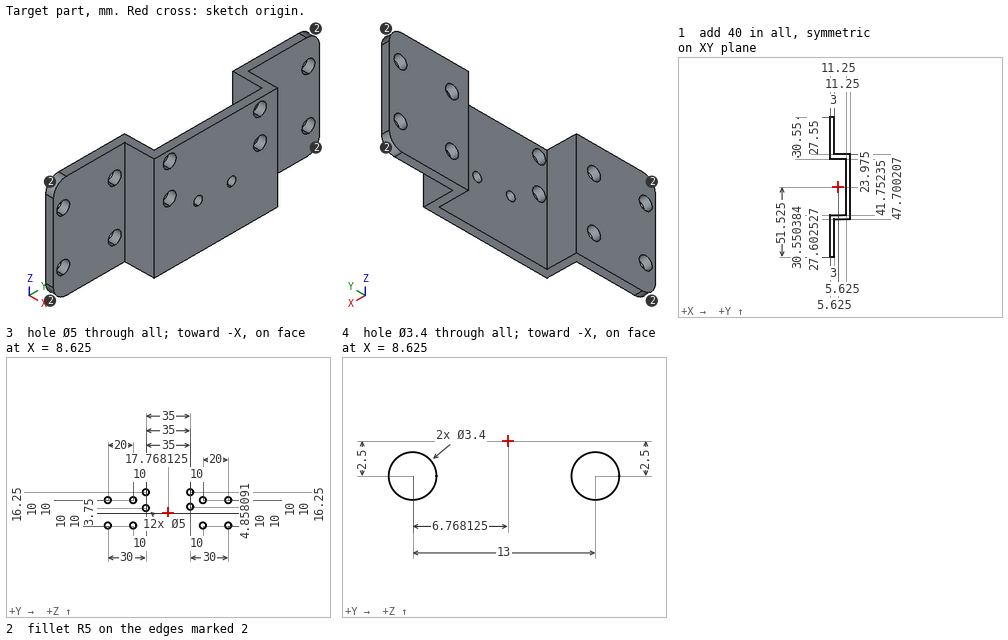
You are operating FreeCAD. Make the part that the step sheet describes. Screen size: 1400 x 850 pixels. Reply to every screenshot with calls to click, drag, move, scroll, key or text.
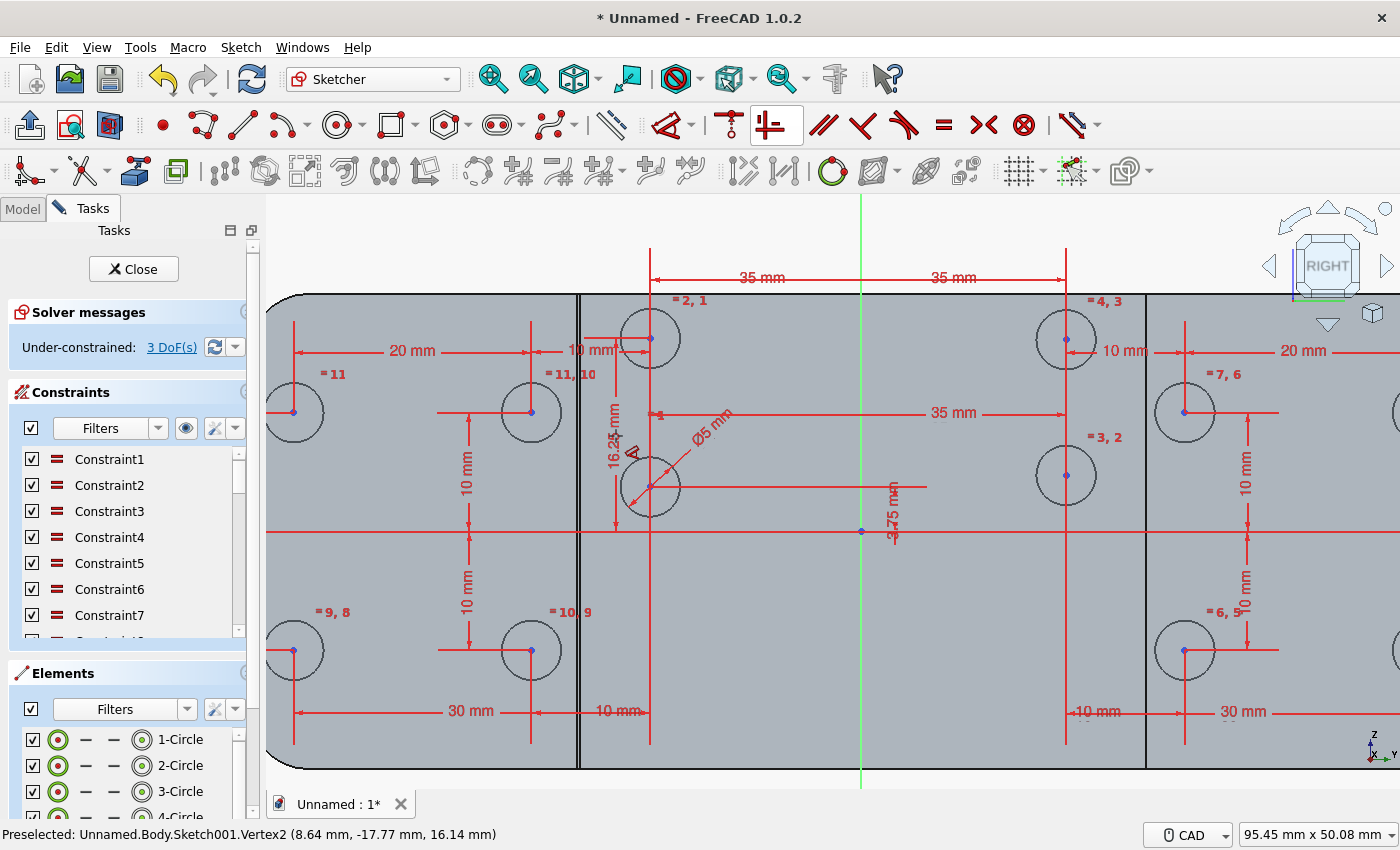
click(1066, 340)
click(1100, 436)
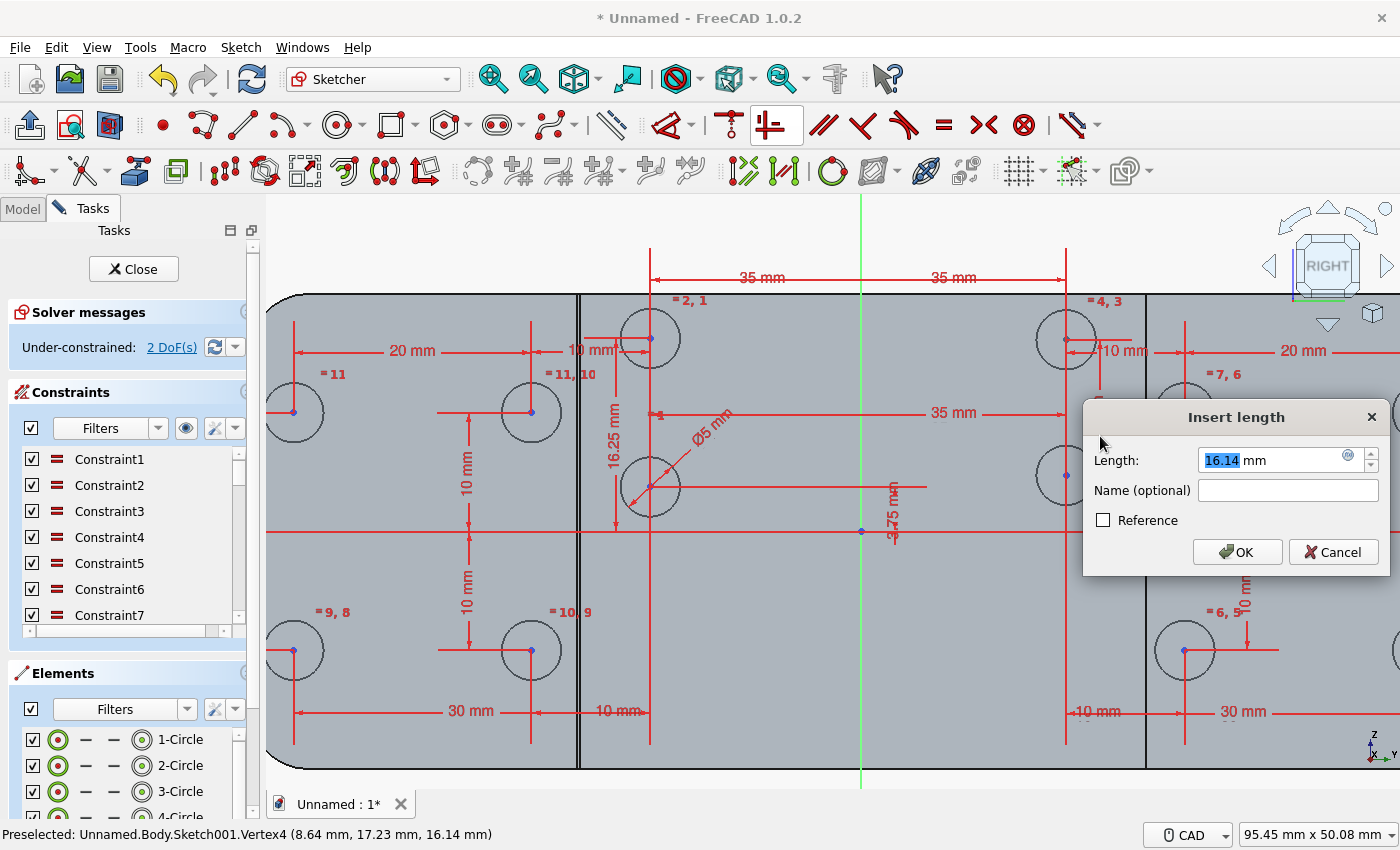
text(16.25)
key(Return)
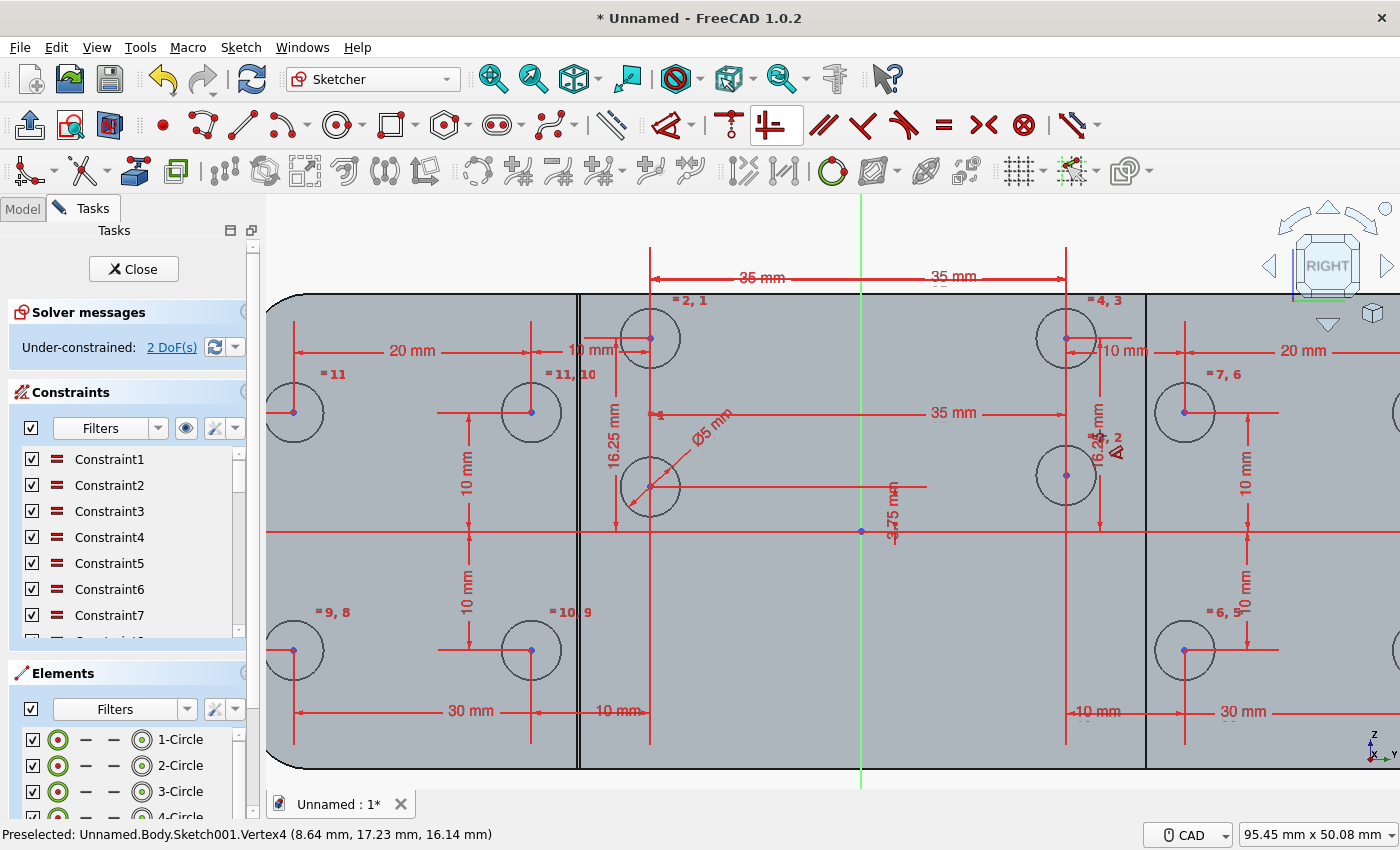
click(1066, 475)
click(1100, 503)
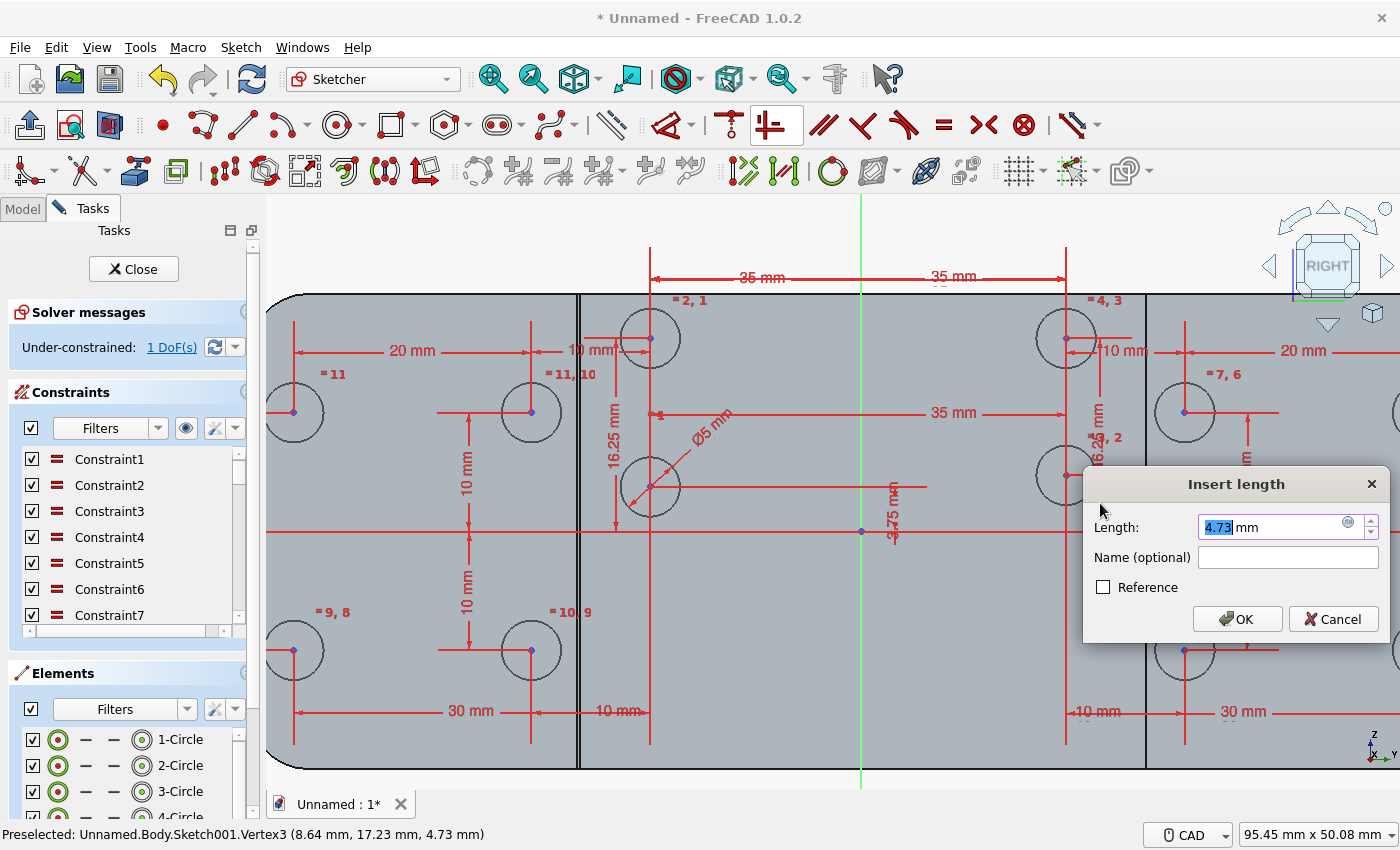
text(4.858091)
key(Return)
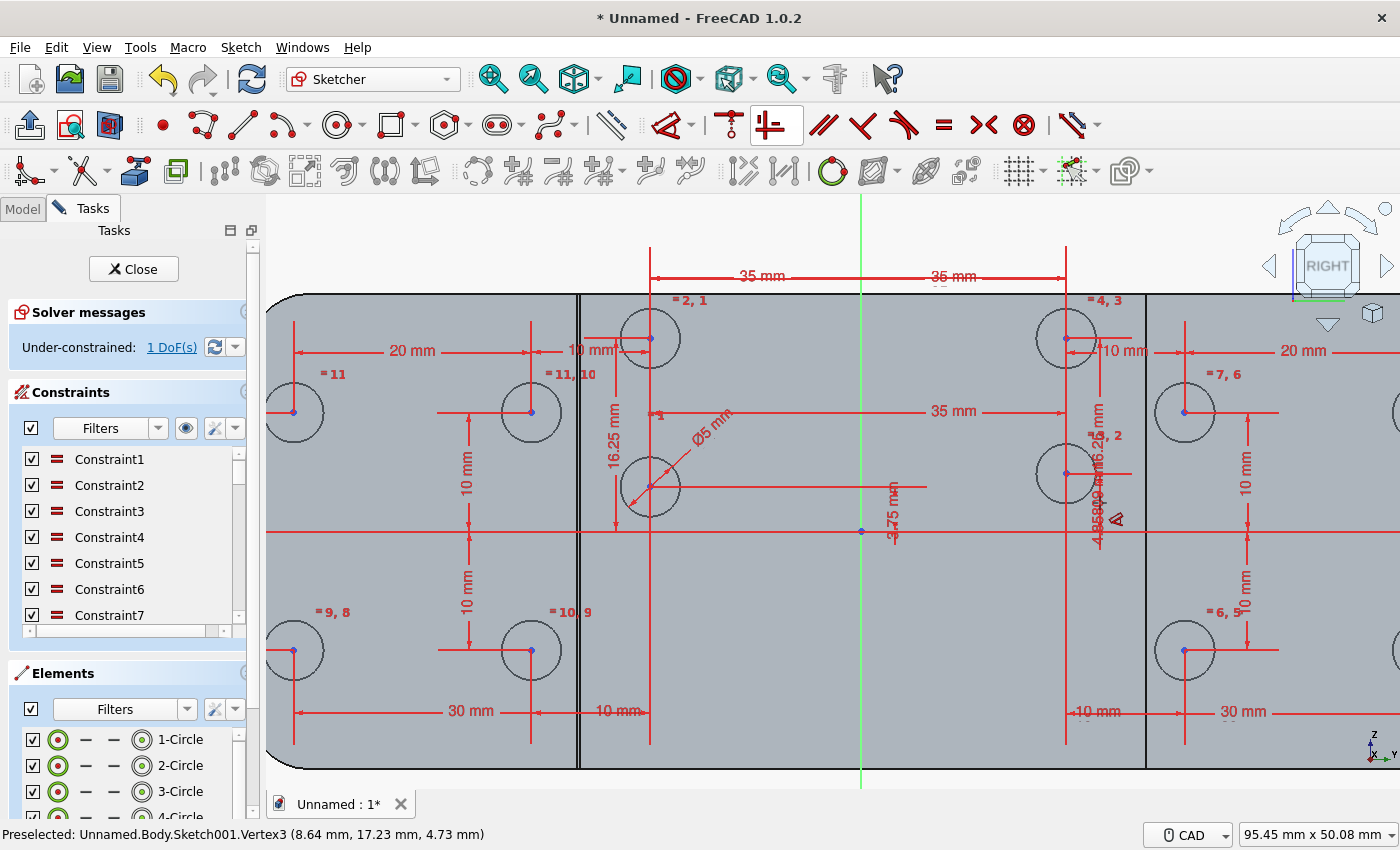
click(650, 487)
click(756, 566)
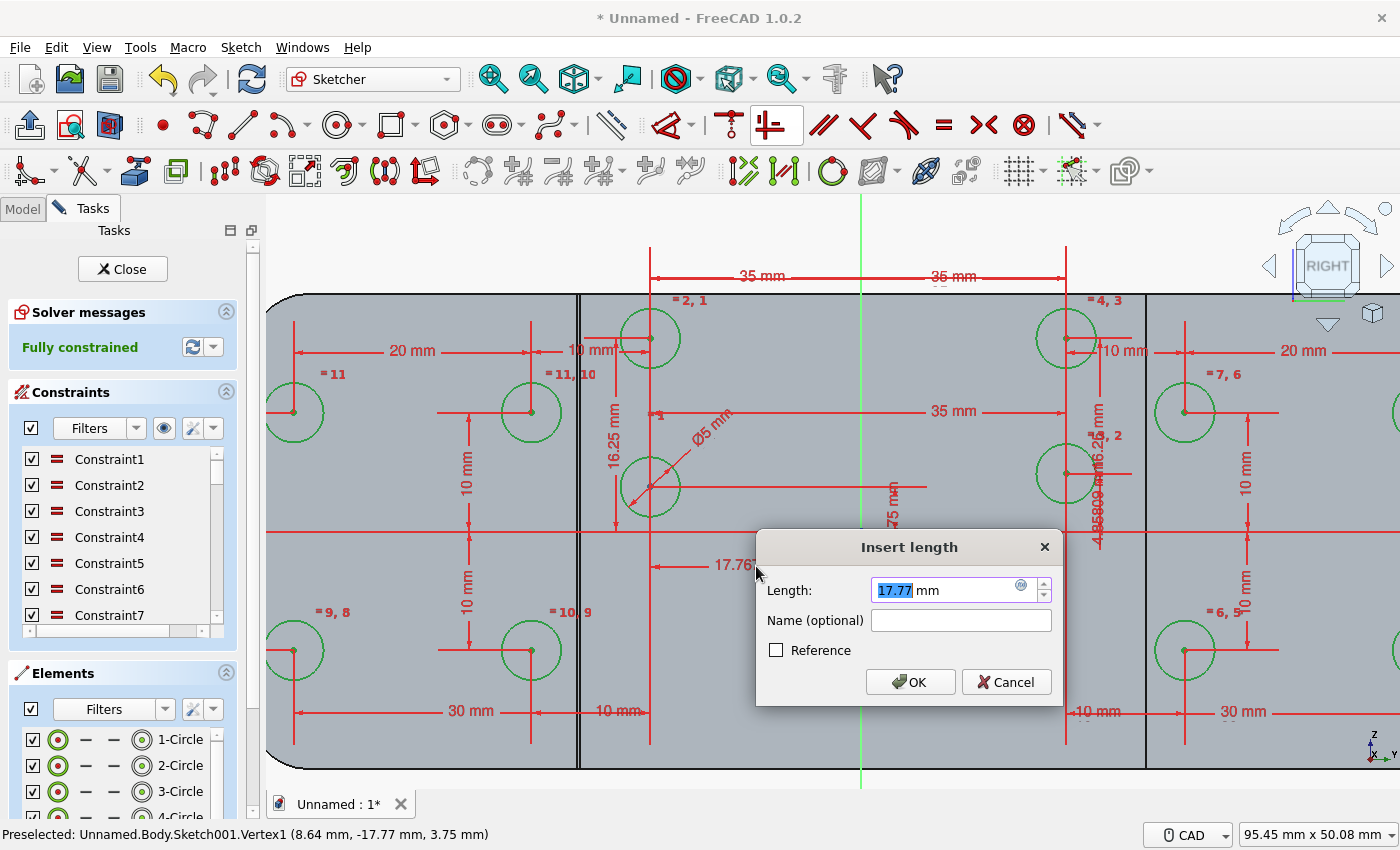
text(17.768125)
key(Return)
key(Escape)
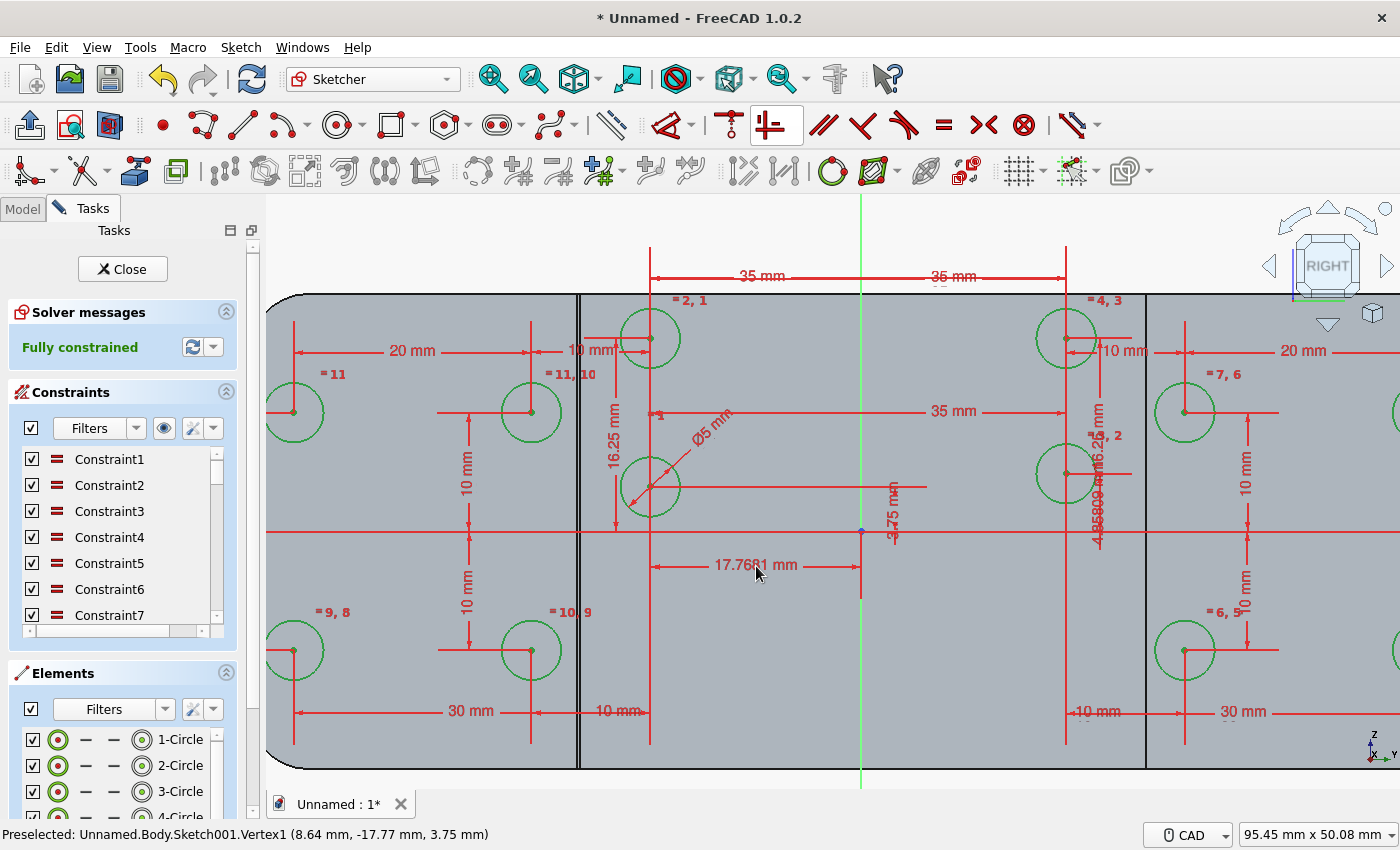
click(123, 269)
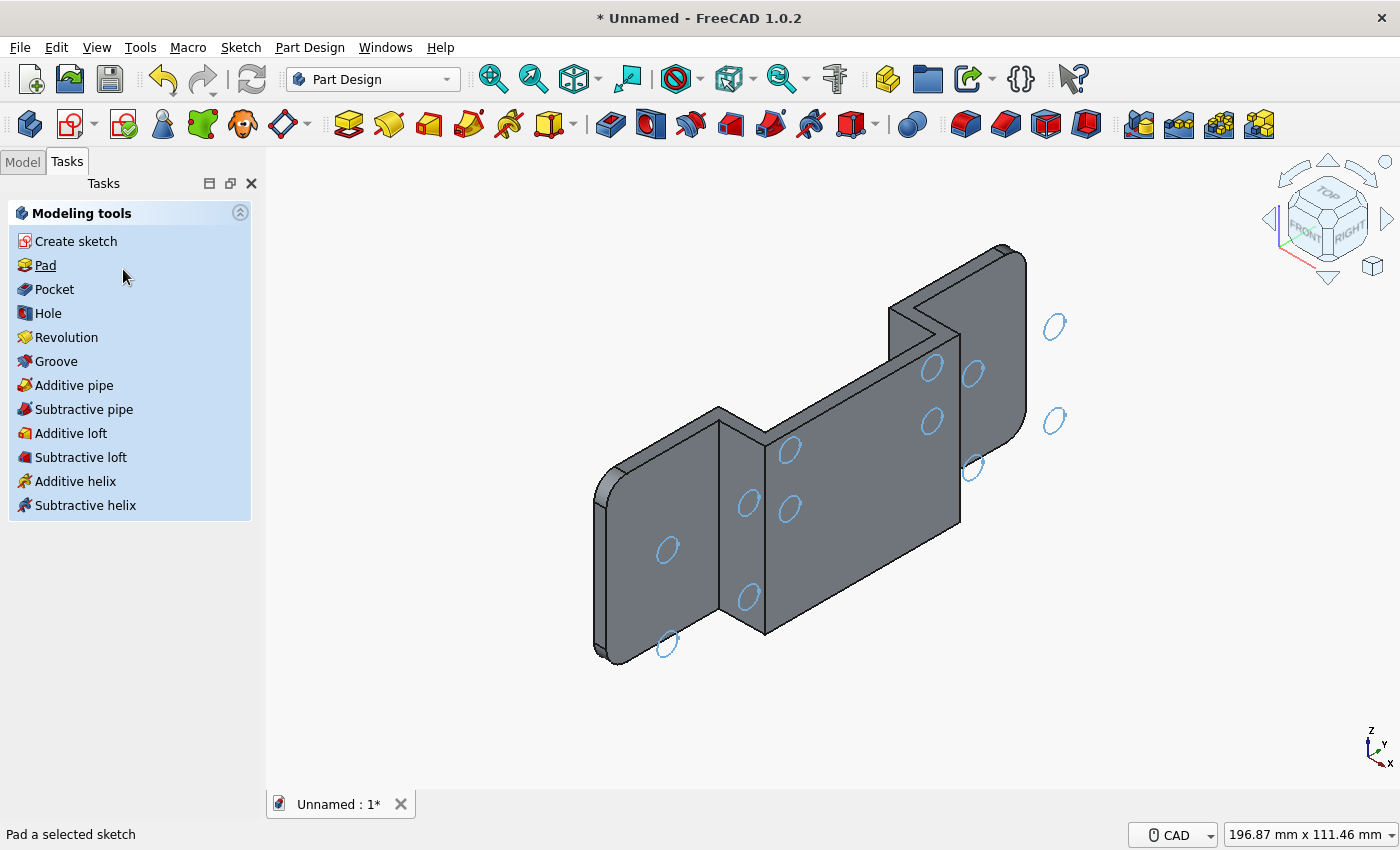
click(652, 124)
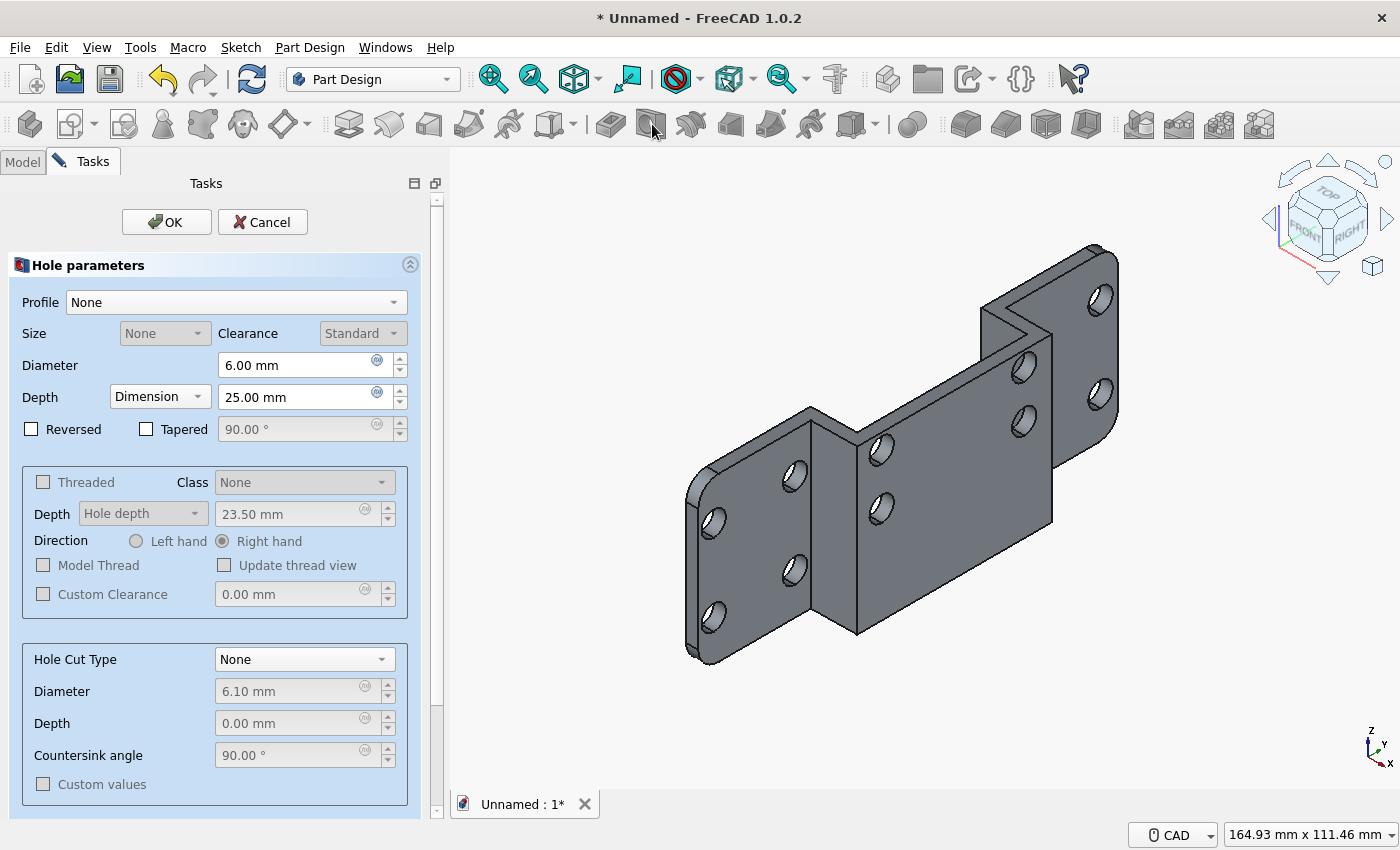
triple_click(305, 365)